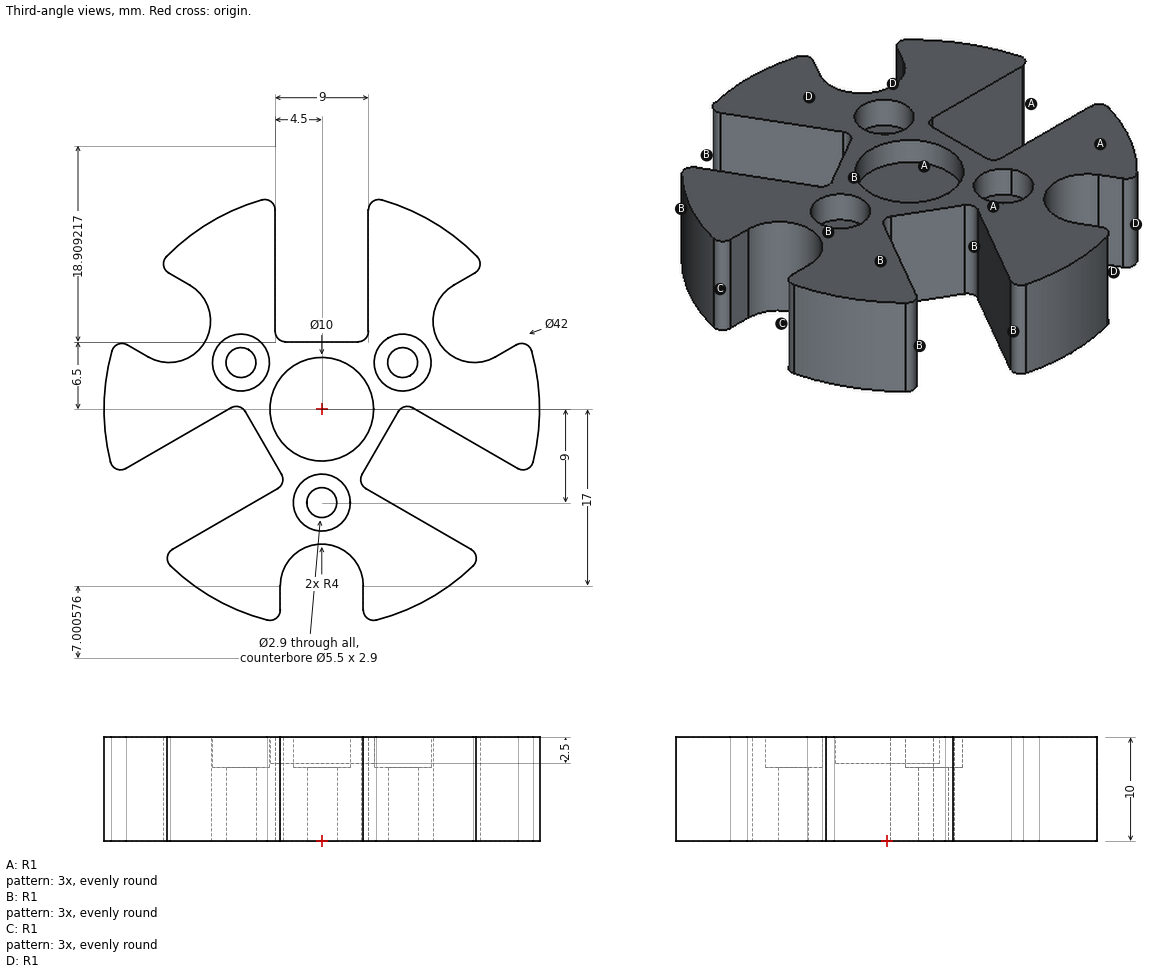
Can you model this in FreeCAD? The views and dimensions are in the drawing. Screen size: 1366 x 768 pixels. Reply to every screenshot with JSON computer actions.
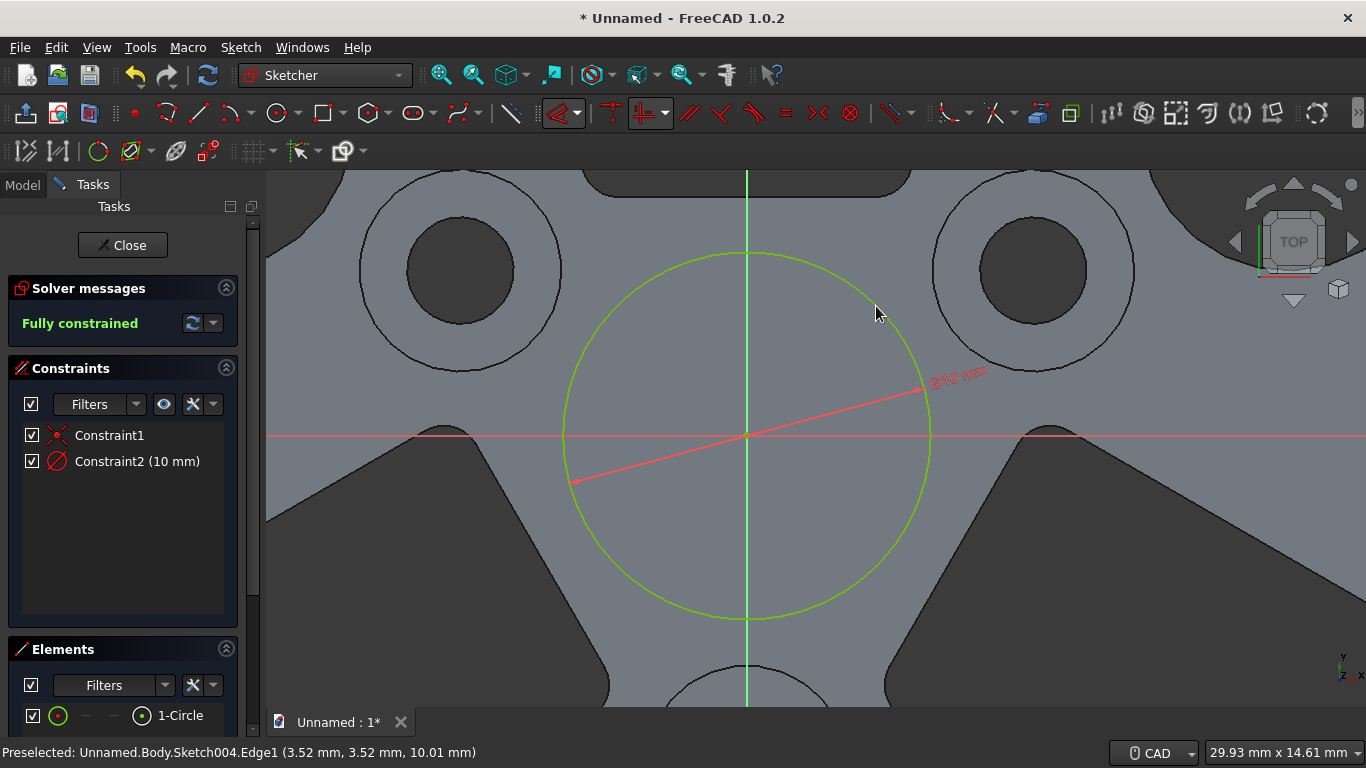
{"action": "left_click", "coordinate": [123, 245]}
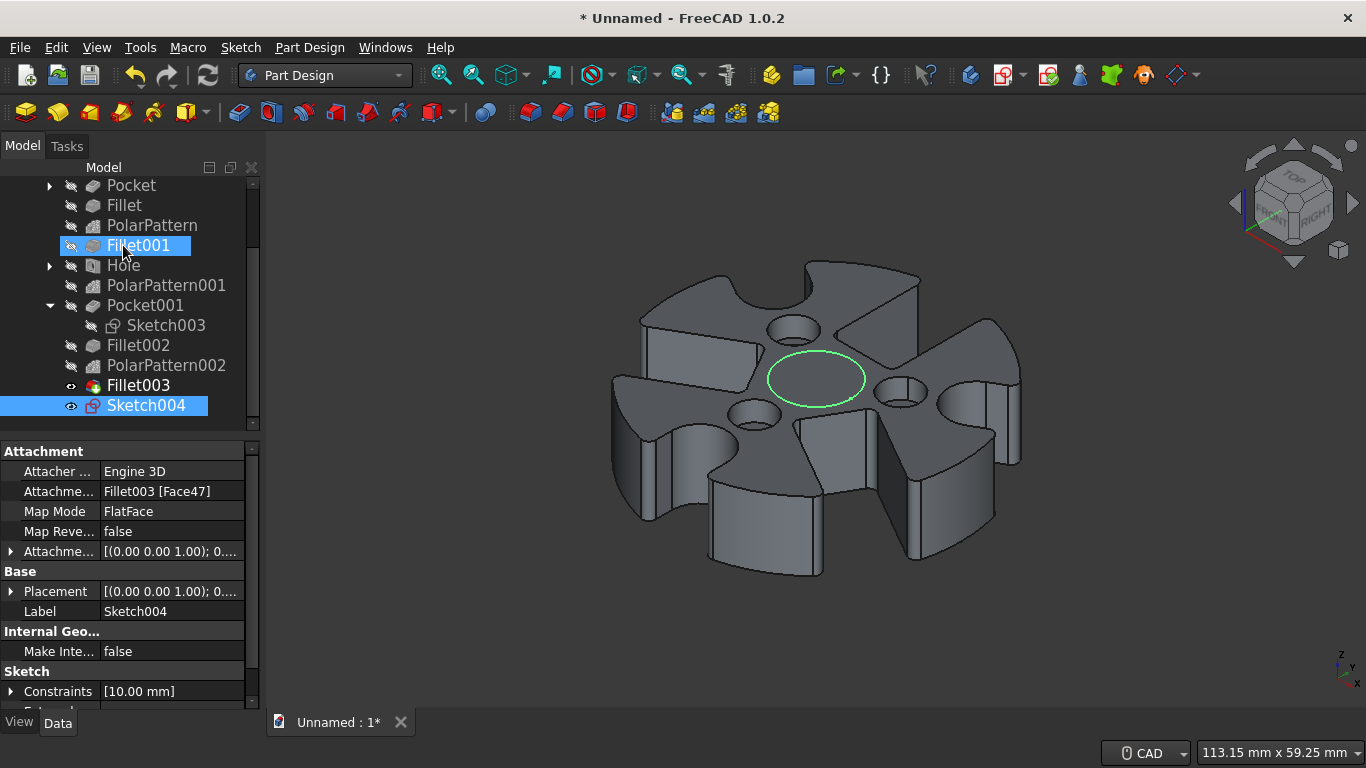
{"action": "left_click", "coordinate": [240, 112]}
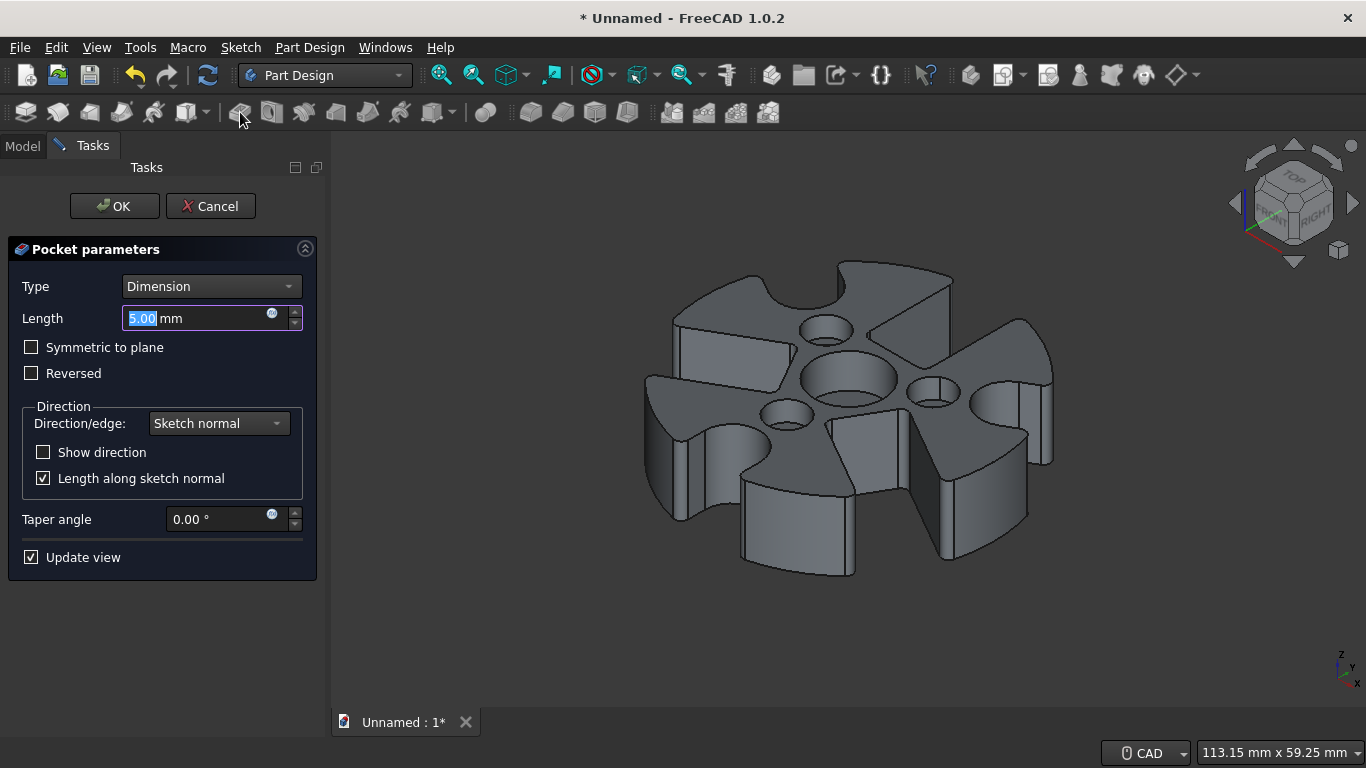
{"action": "type", "text": "2.5"}
{"action": "key", "text": "Tab"}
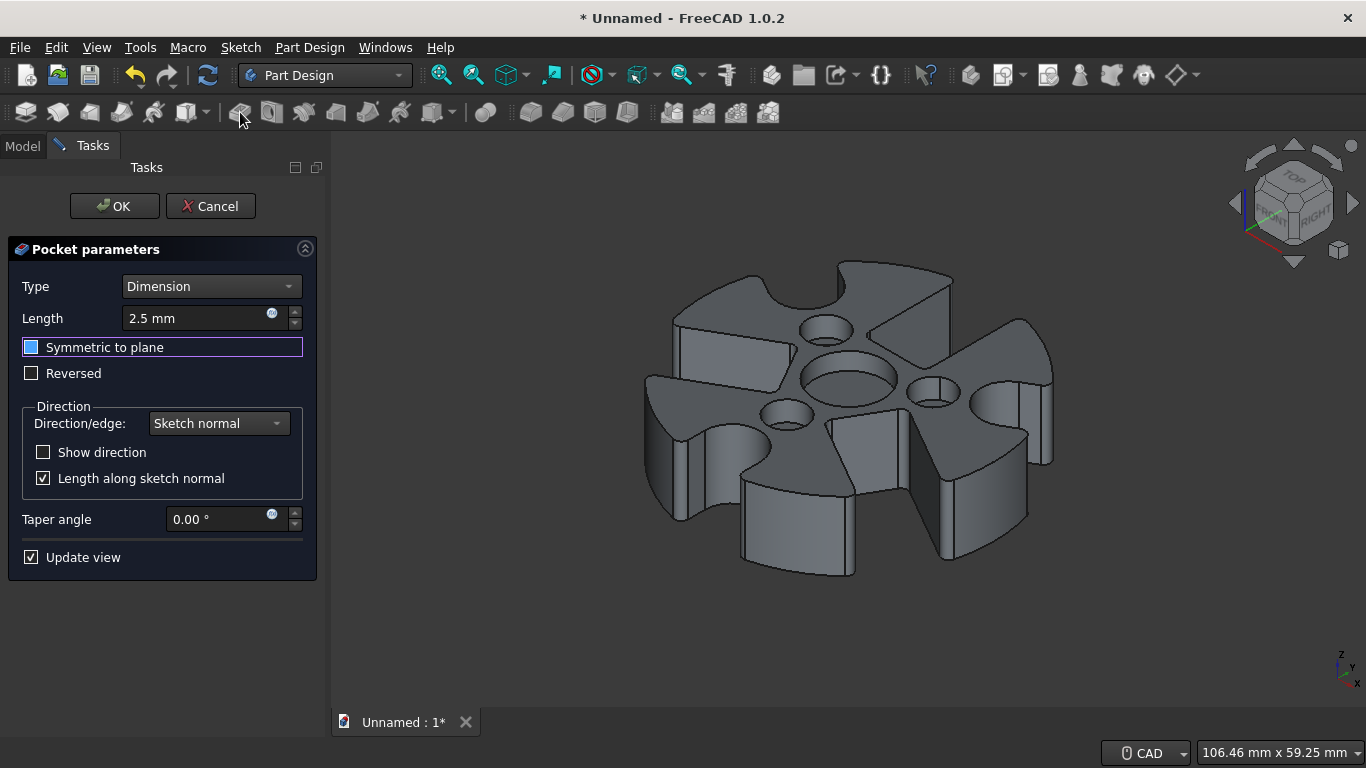
{"action": "left_click", "coordinate": [115, 206]}